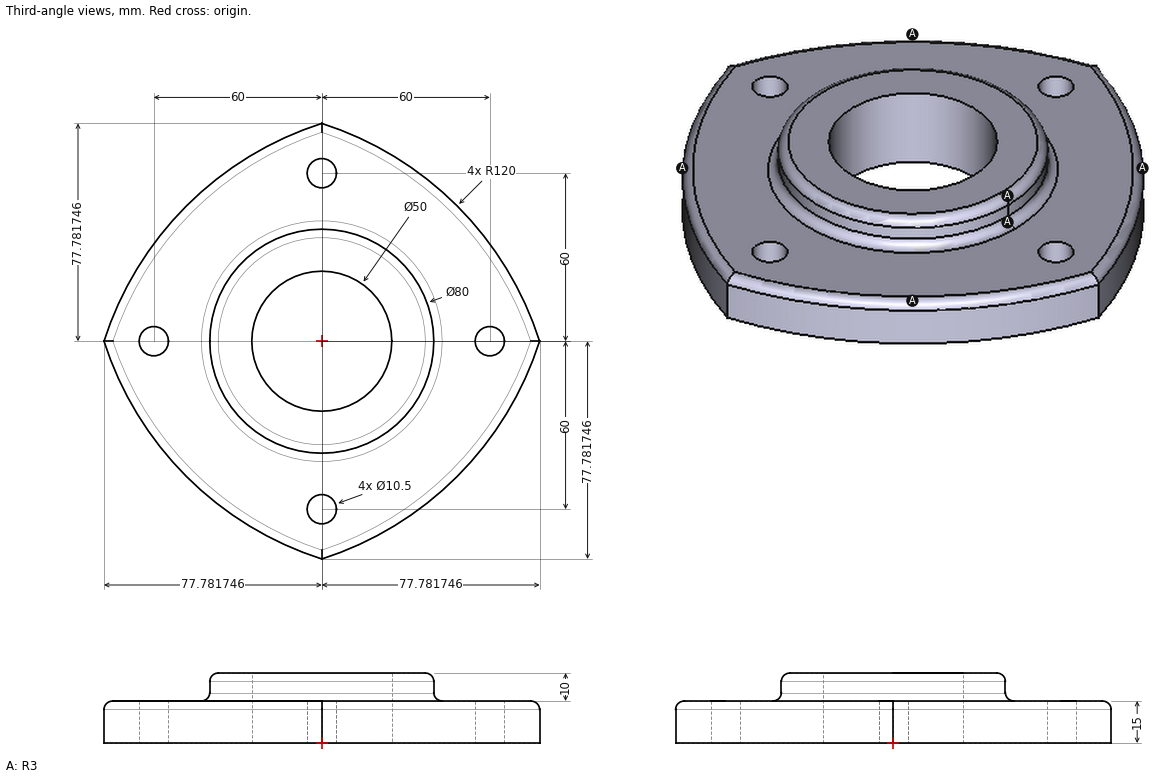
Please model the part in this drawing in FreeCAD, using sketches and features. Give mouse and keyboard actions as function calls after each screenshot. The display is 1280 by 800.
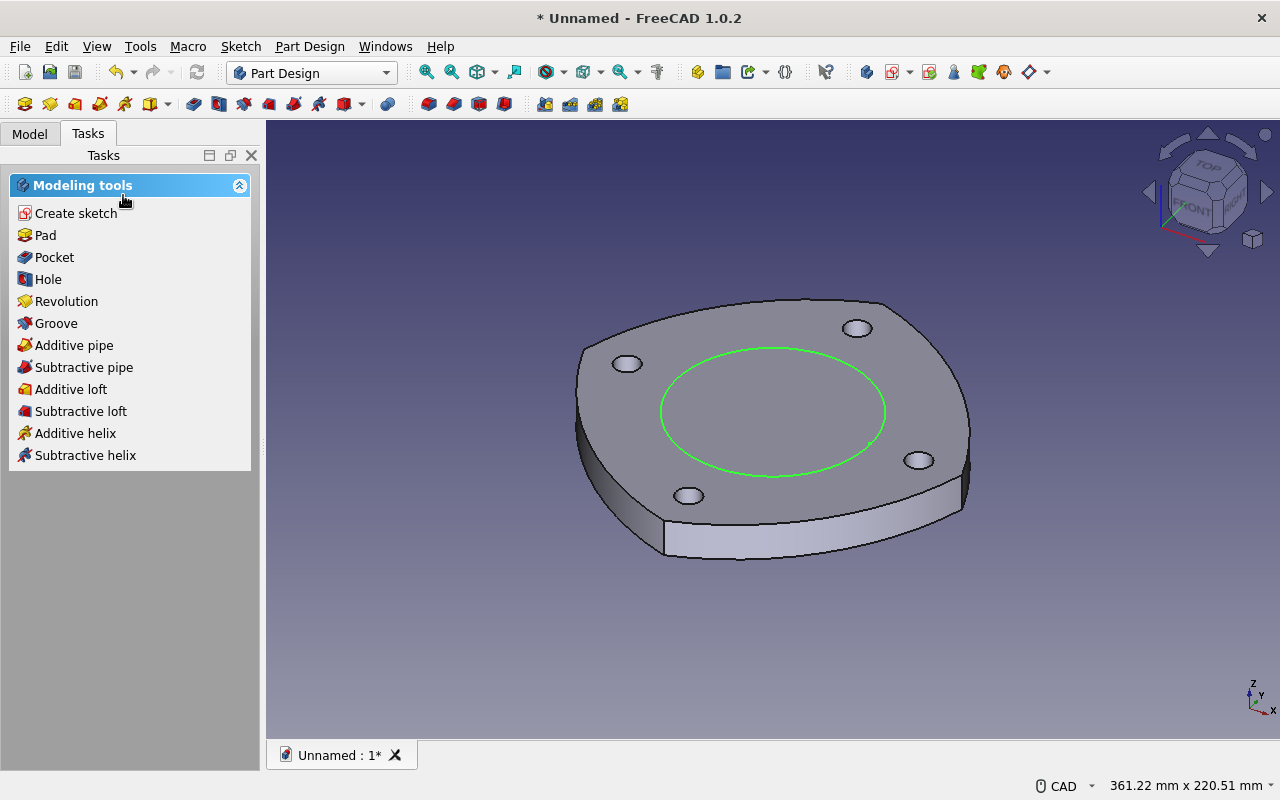
click(25, 104)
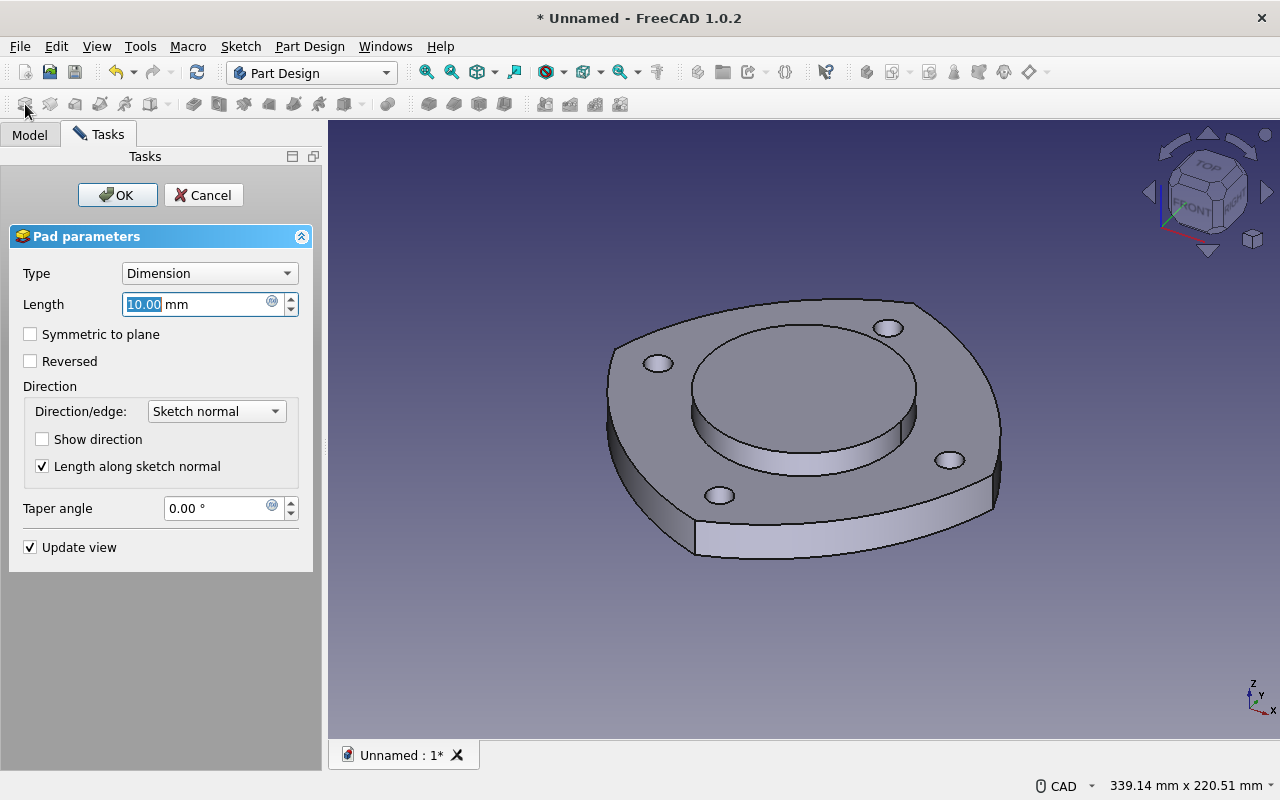
text(10)
key(Tab)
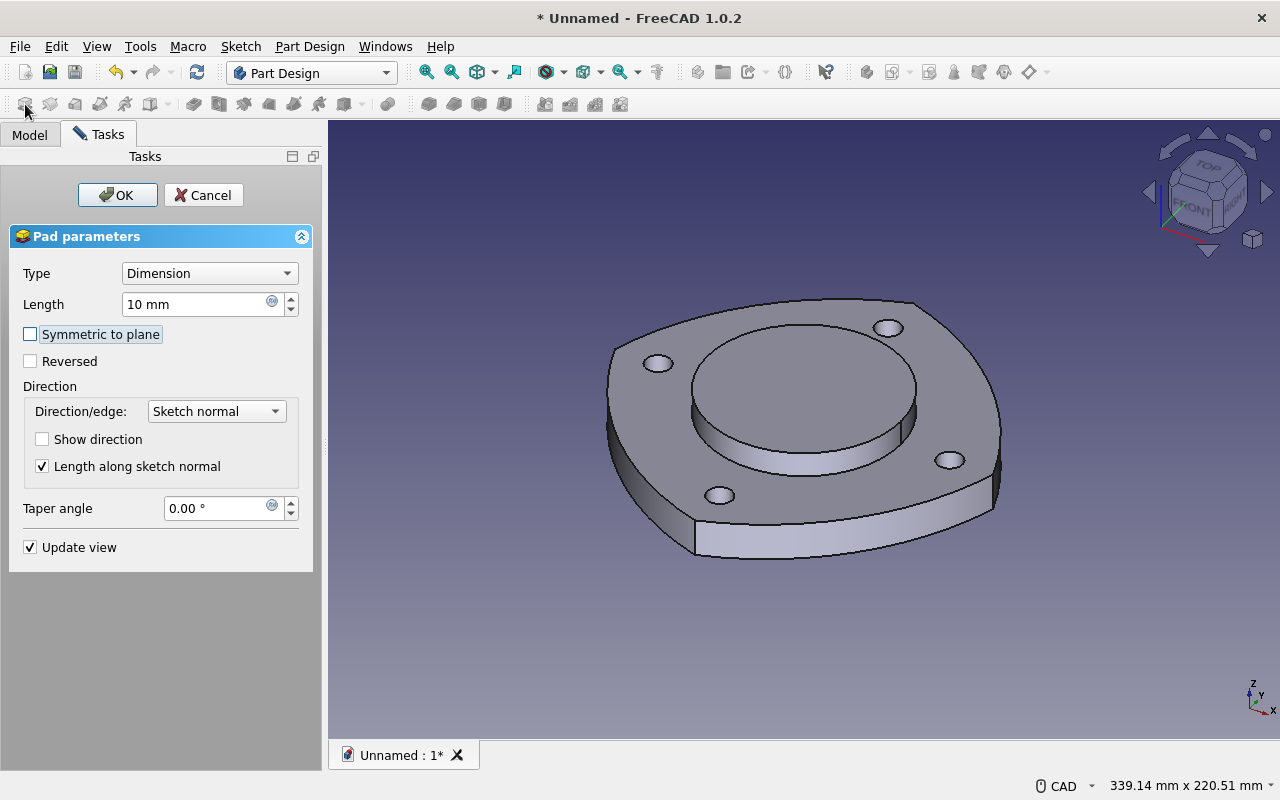
click(118, 195)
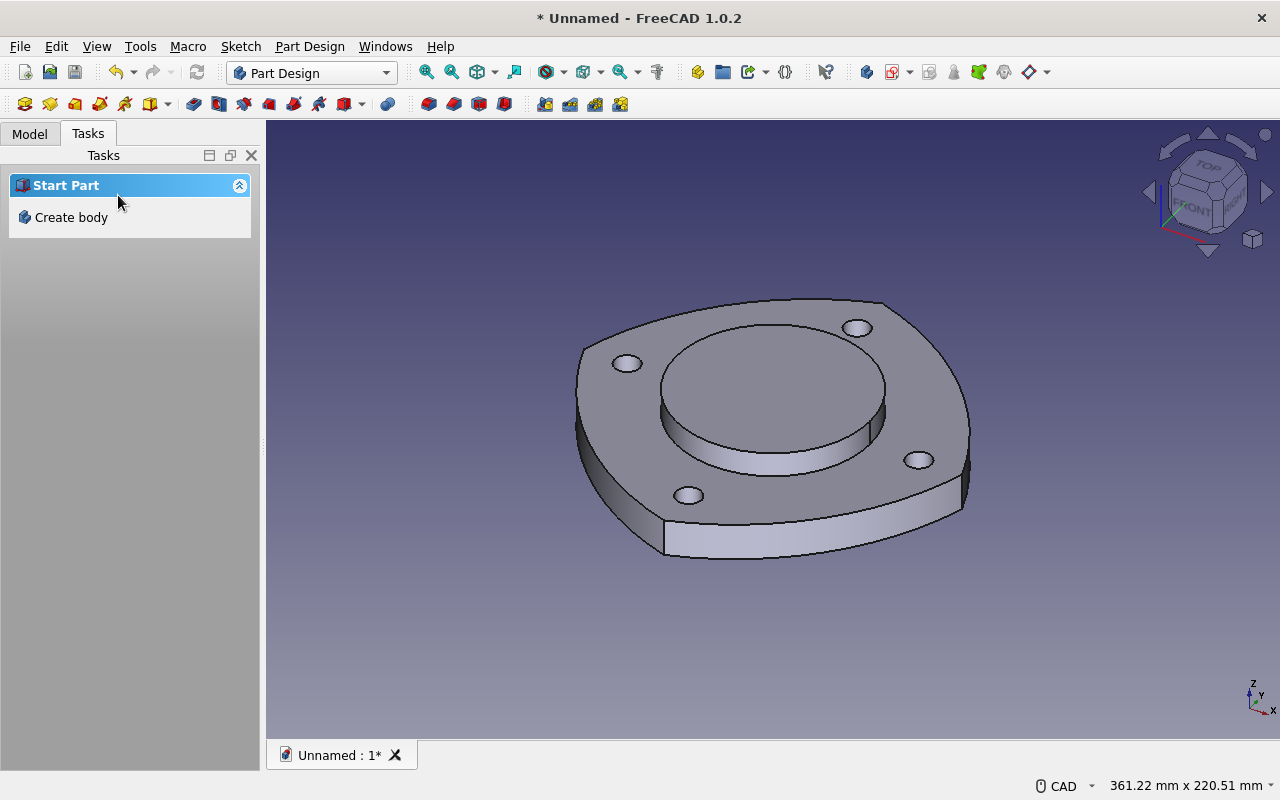
click(773, 388)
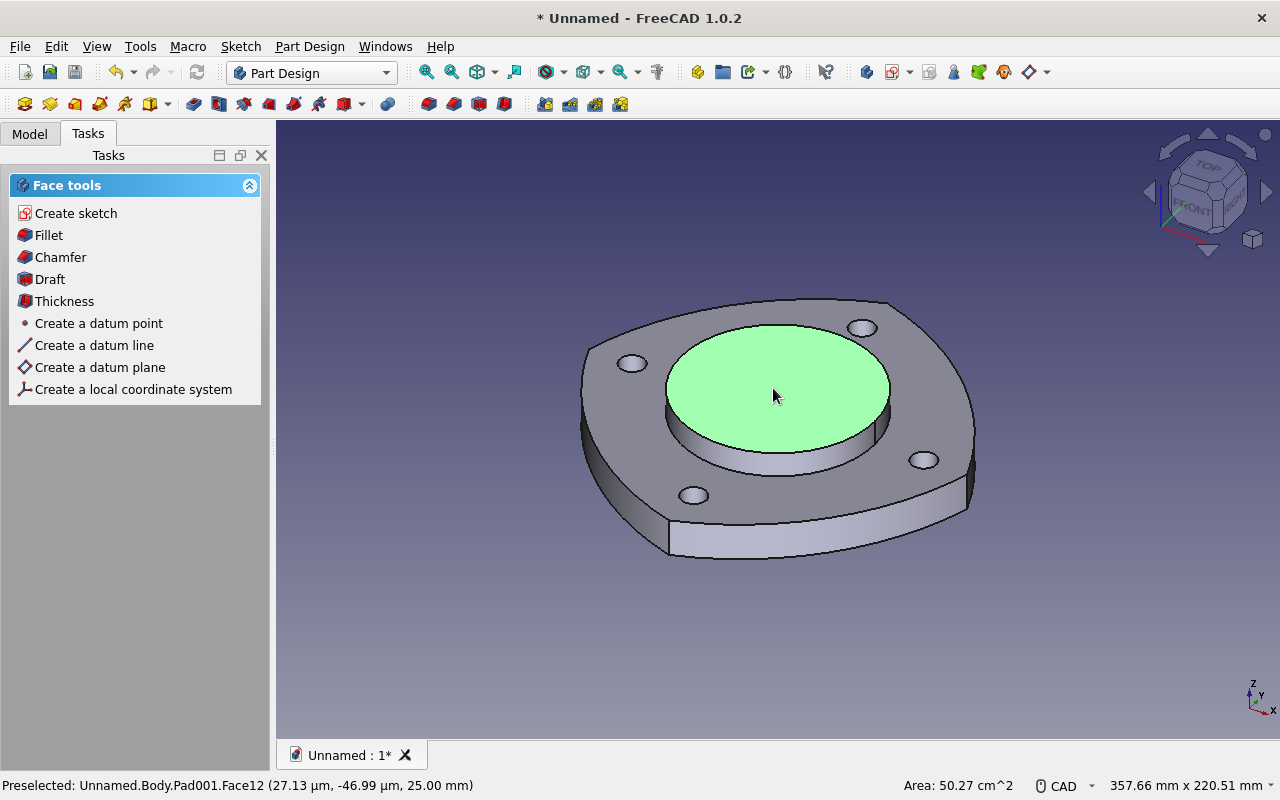
click(892, 72)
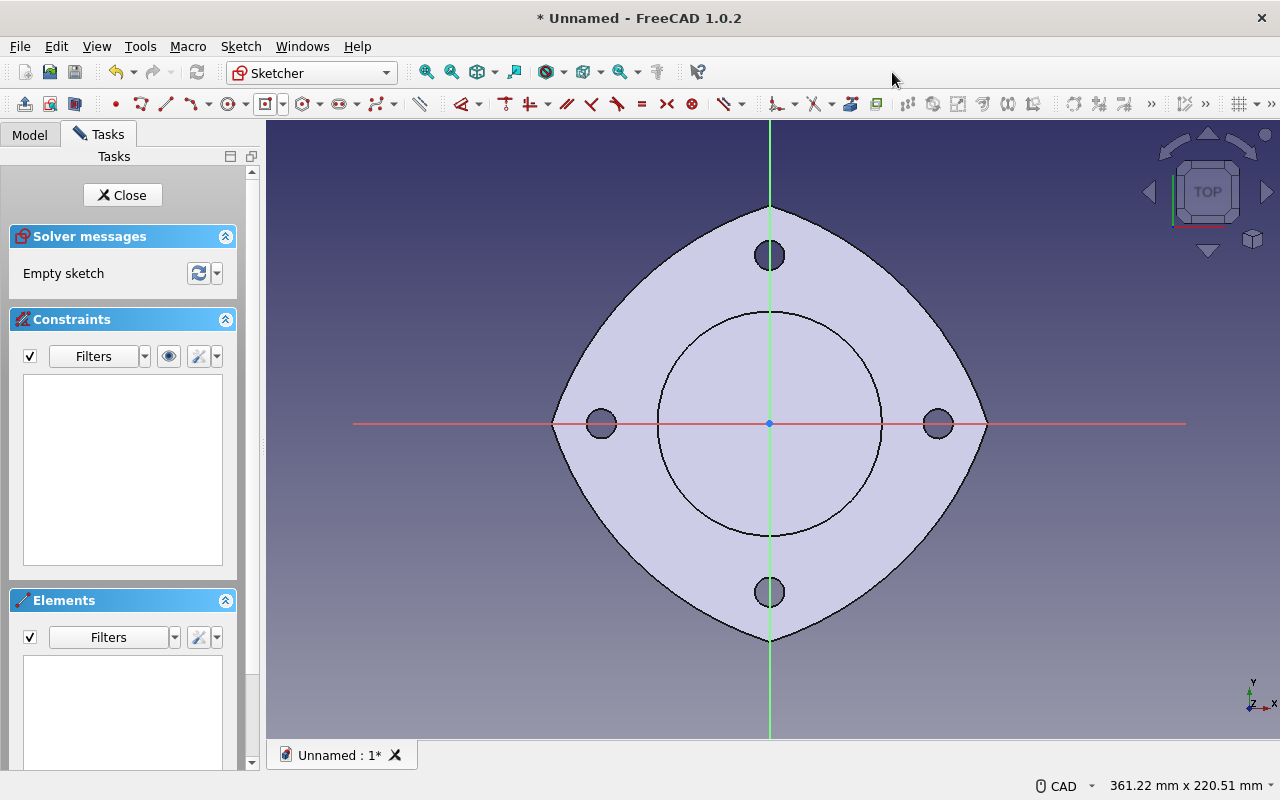
scroll(808, 420, up, 5)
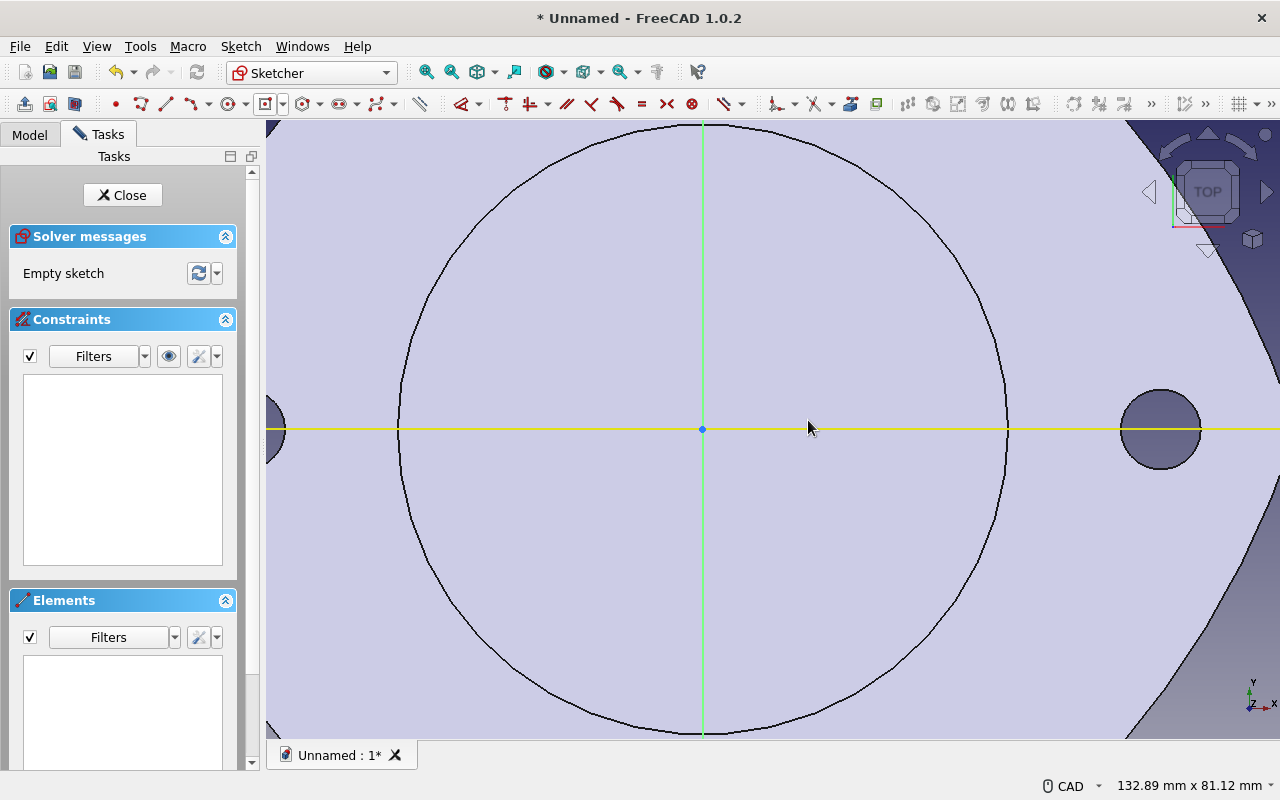
click(228, 104)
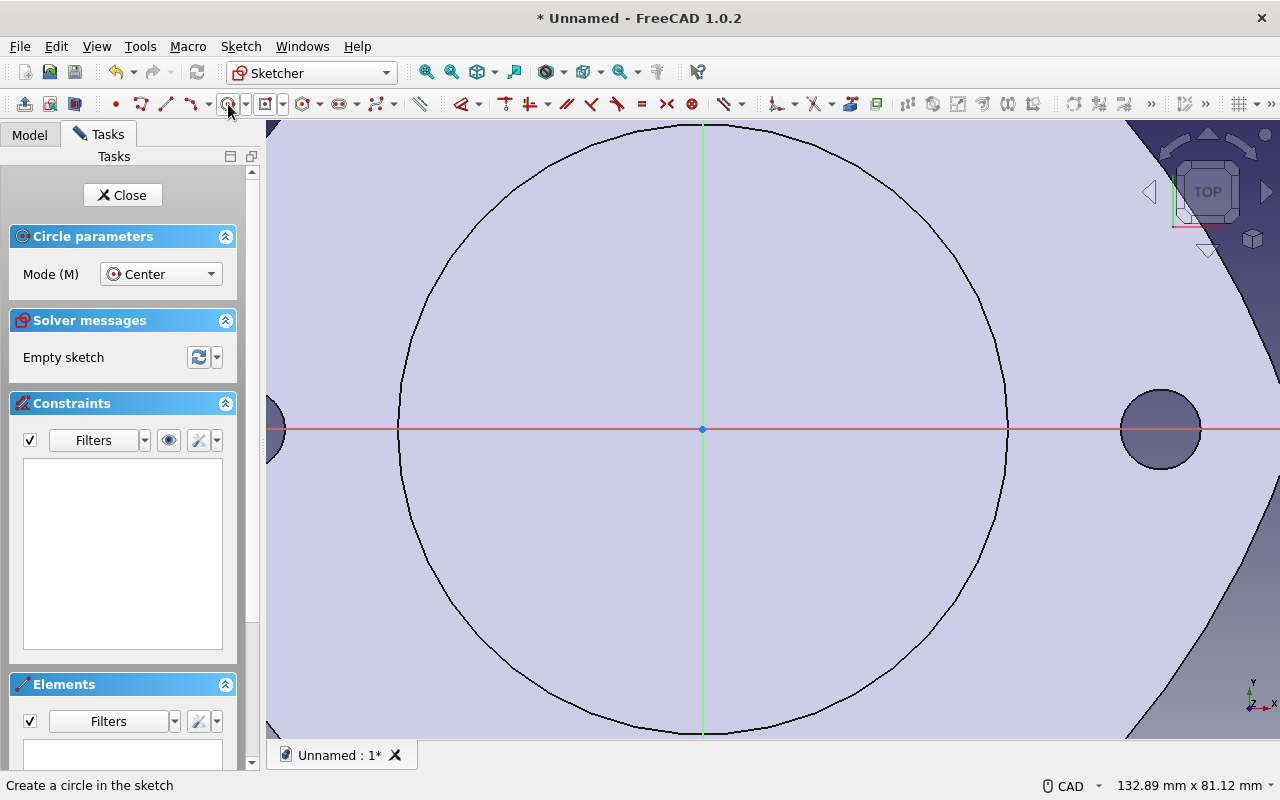
click(703, 429)
click(838, 295)
key(Escape)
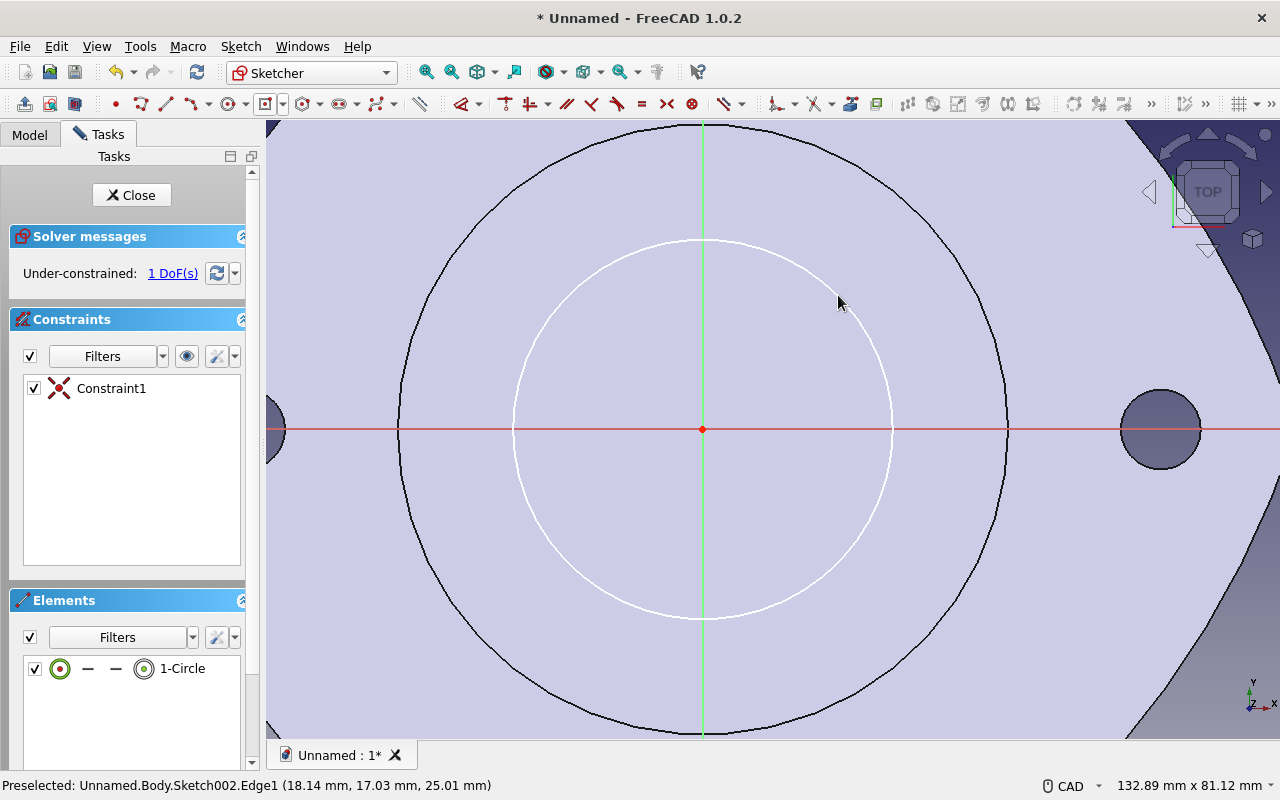
key(d)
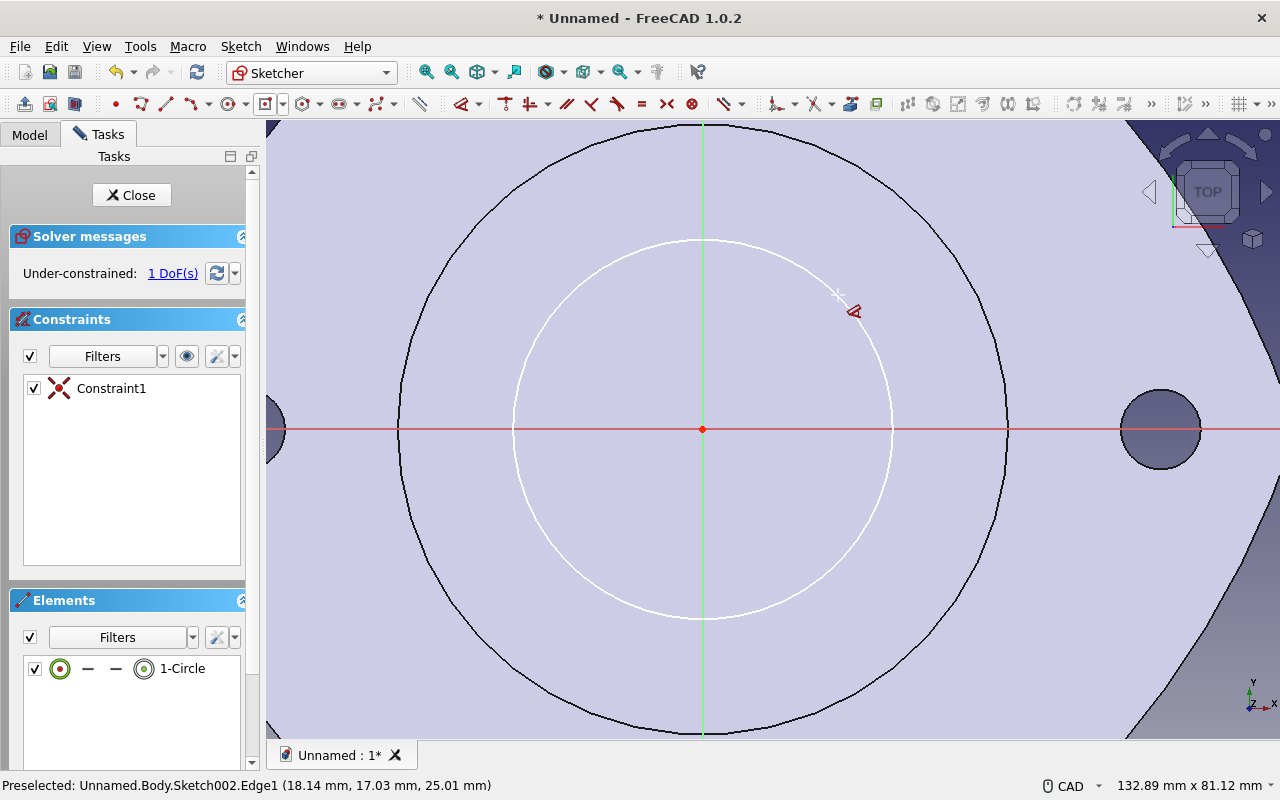
click(837, 295)
click(860, 272)